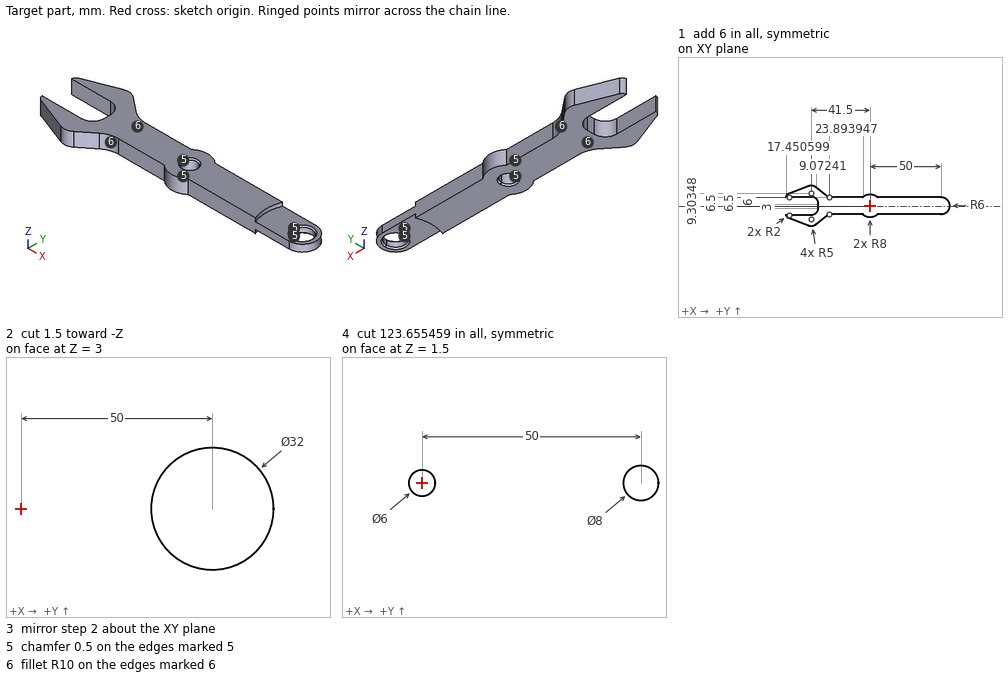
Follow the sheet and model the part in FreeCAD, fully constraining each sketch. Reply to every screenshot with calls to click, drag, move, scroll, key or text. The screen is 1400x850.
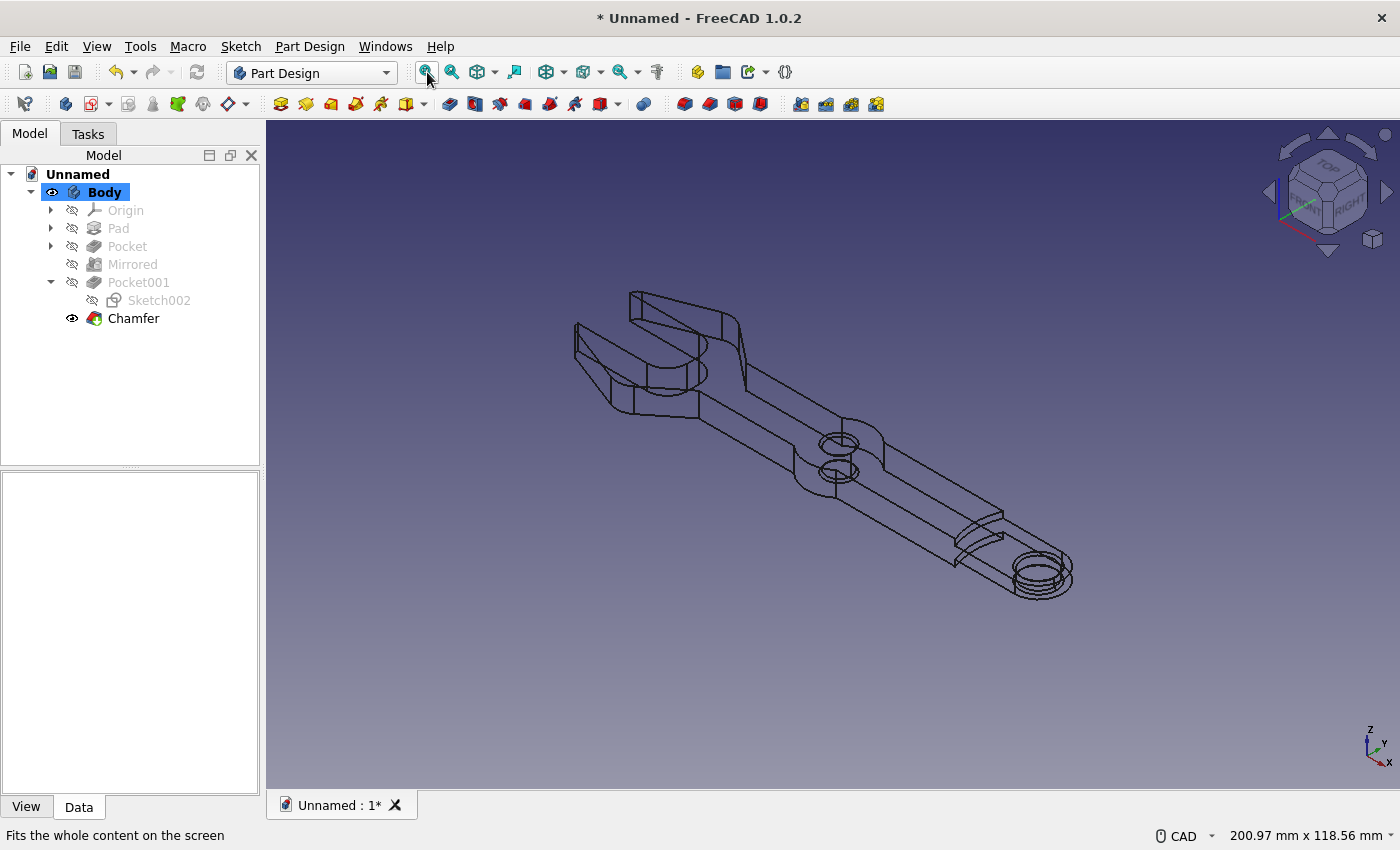
click(746, 376)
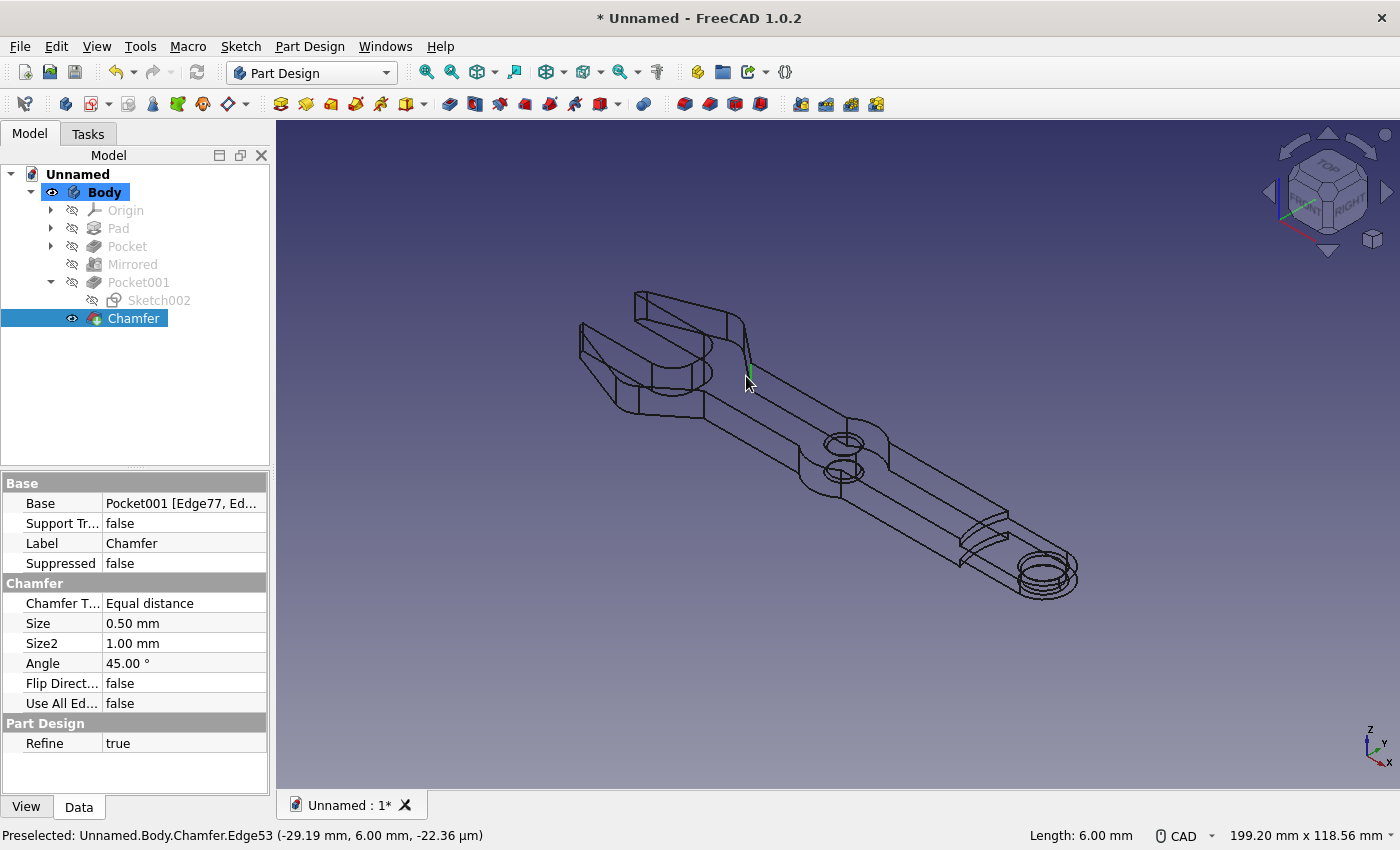
click(704, 404, ctrl)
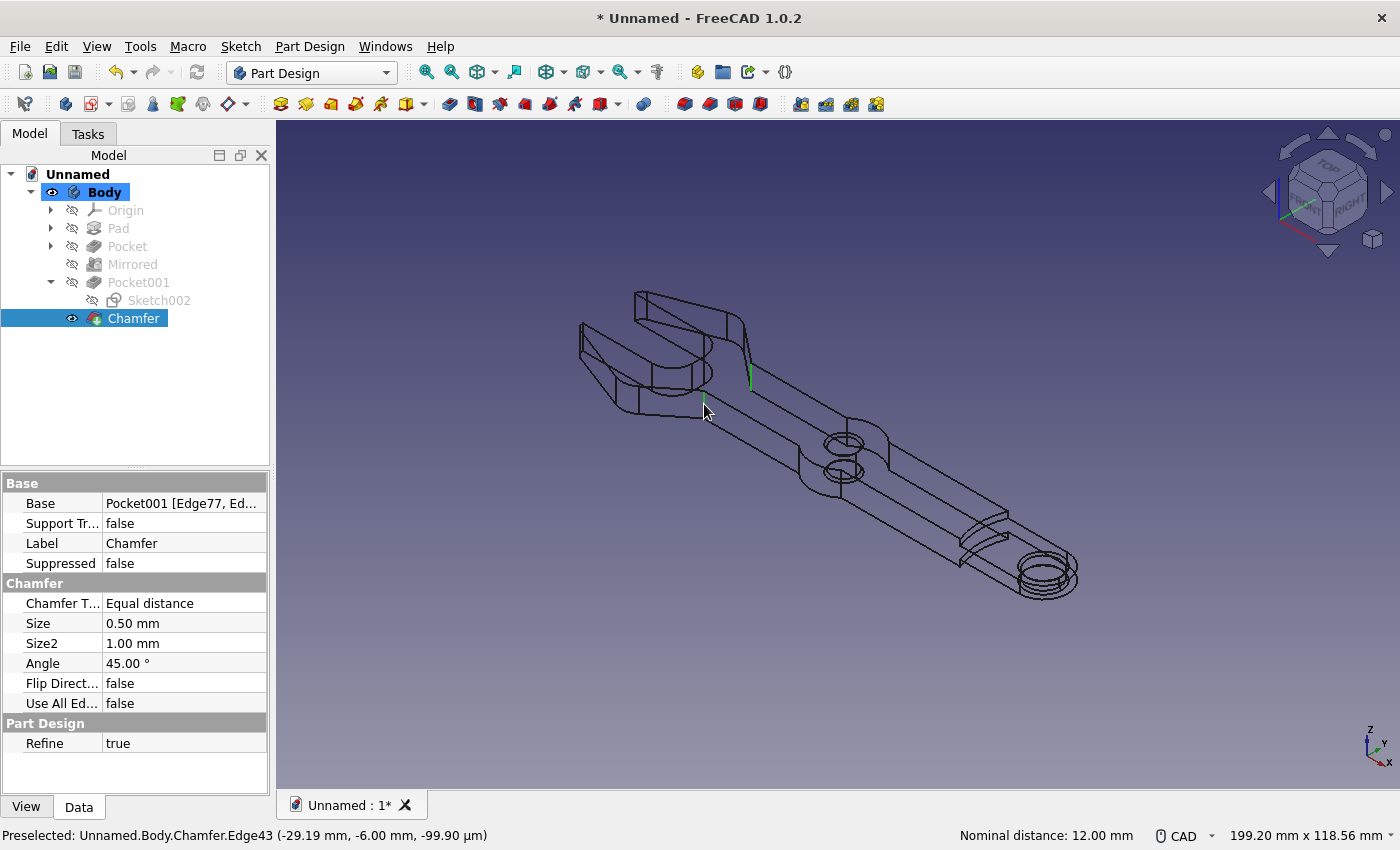
key(v)
key(1)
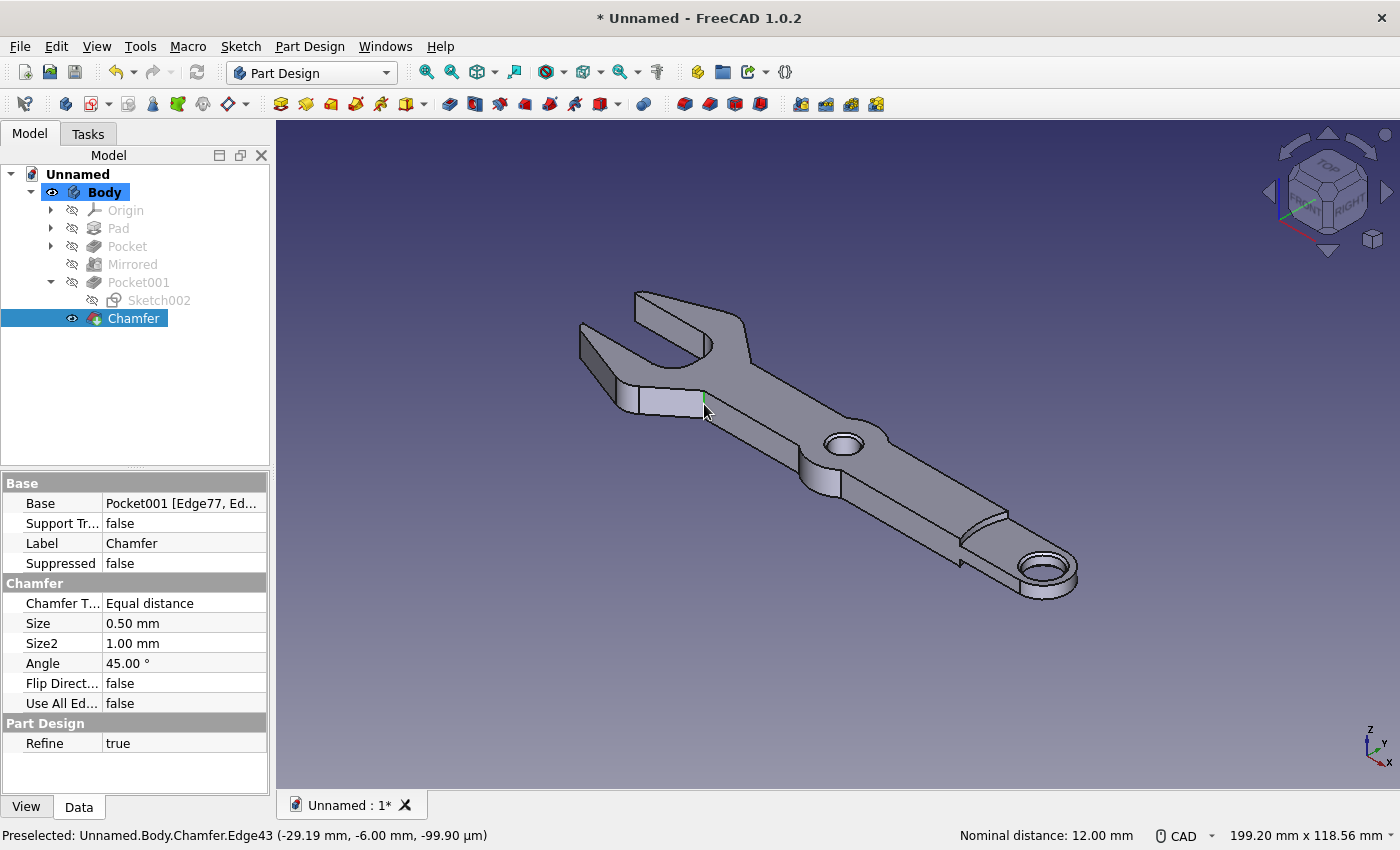
click(685, 104)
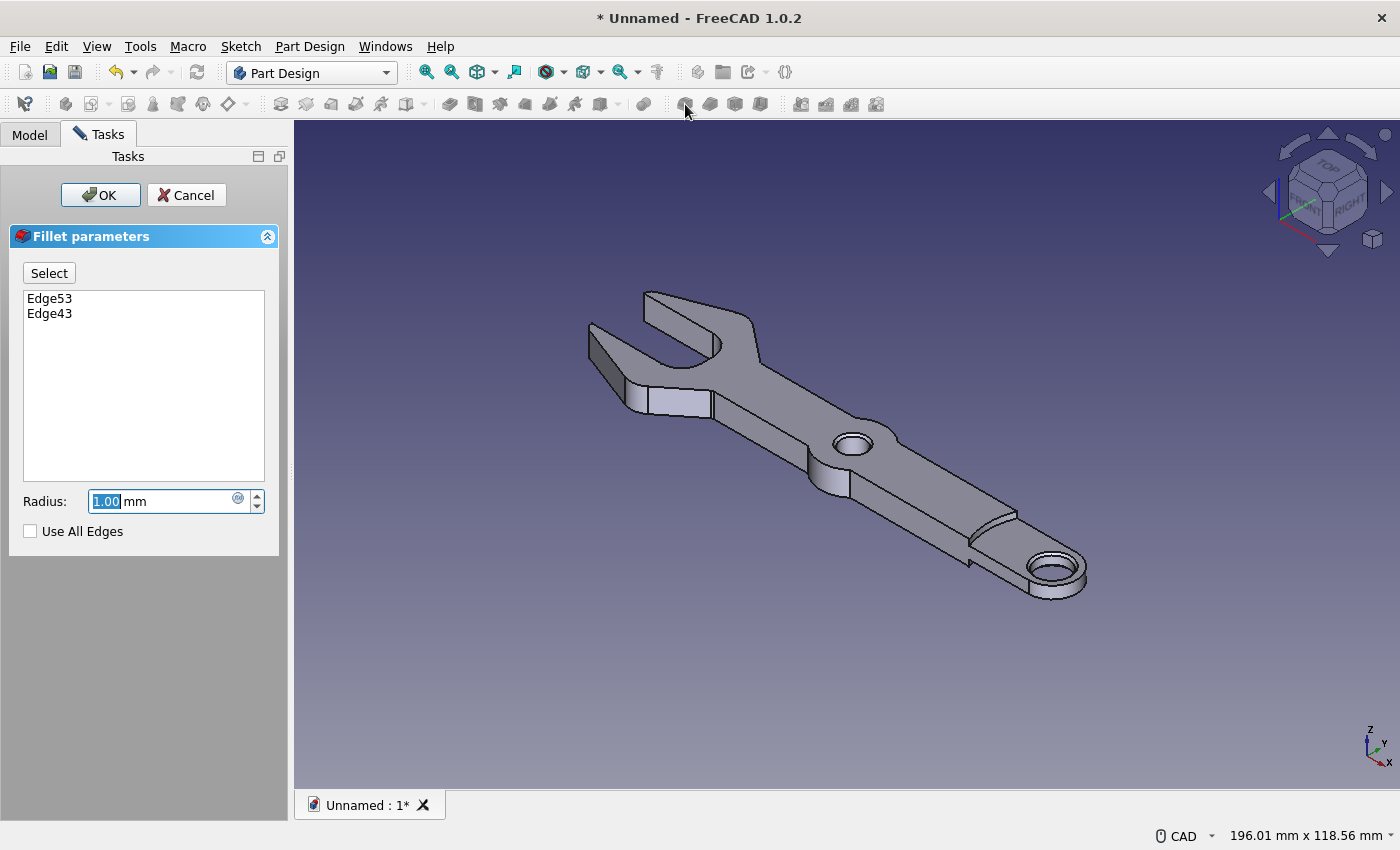
text(10)
key(Tab)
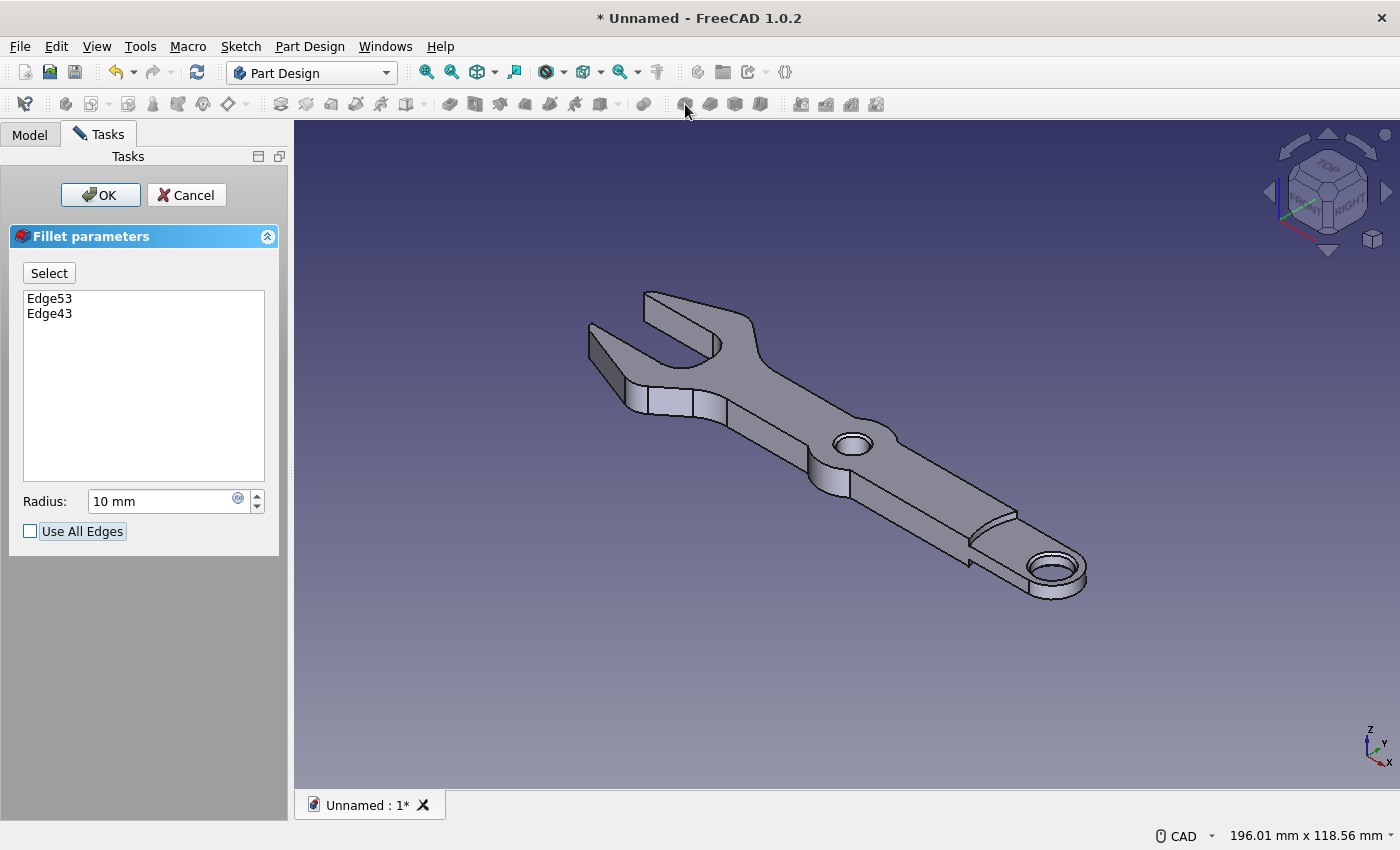
click(101, 195)